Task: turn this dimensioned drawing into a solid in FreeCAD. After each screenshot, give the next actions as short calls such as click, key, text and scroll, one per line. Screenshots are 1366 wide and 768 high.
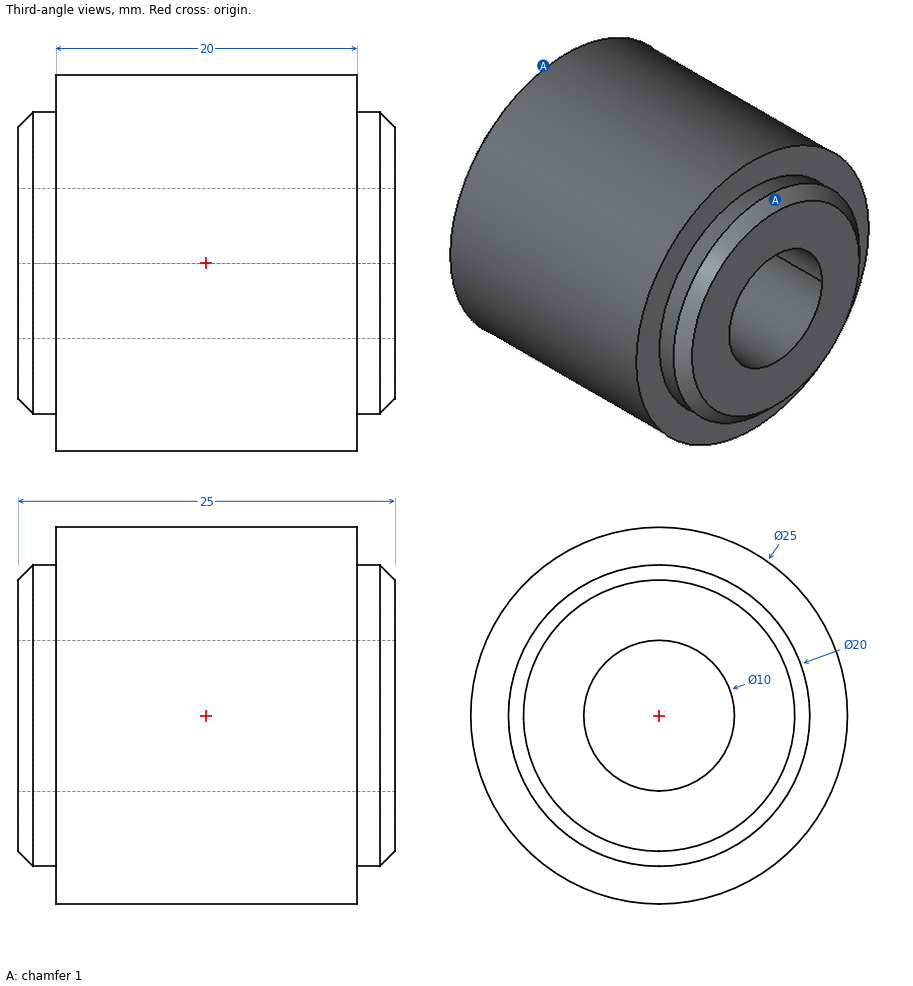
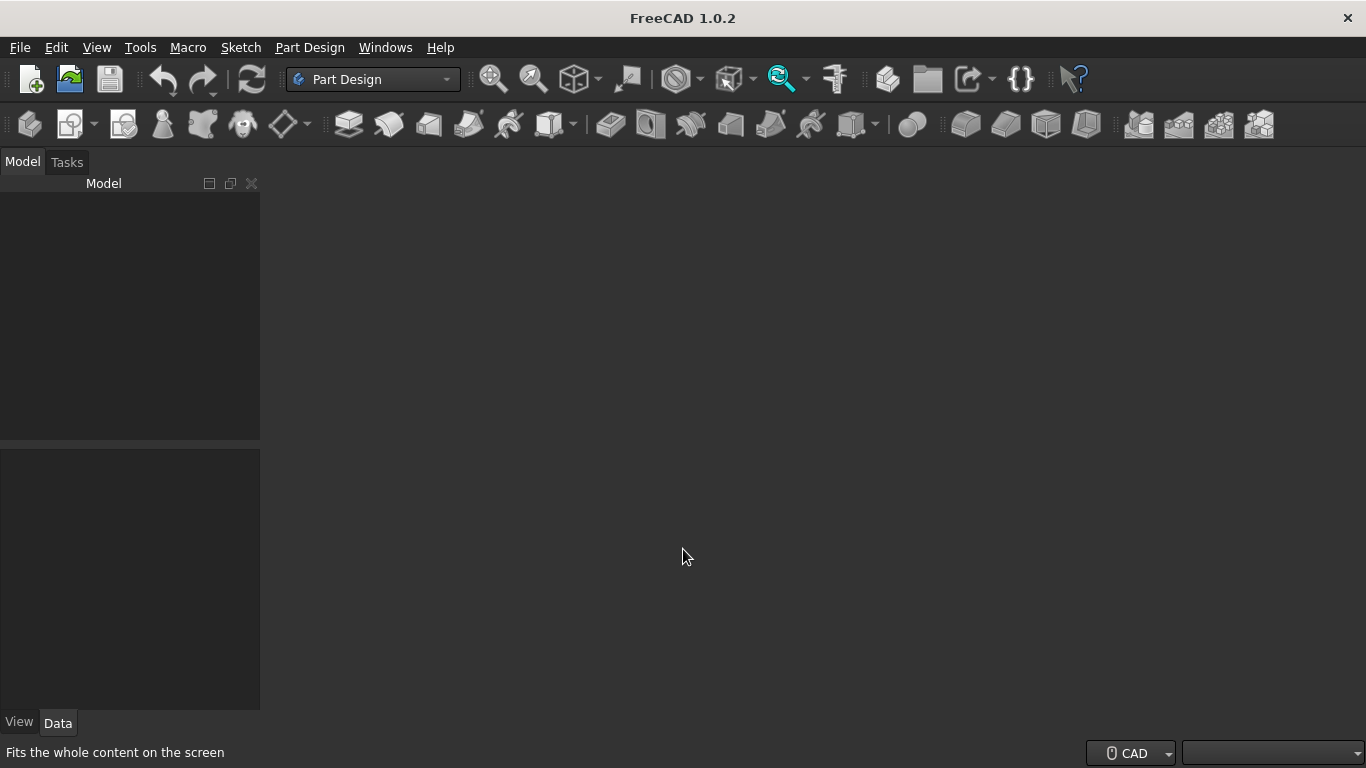
click(30, 80)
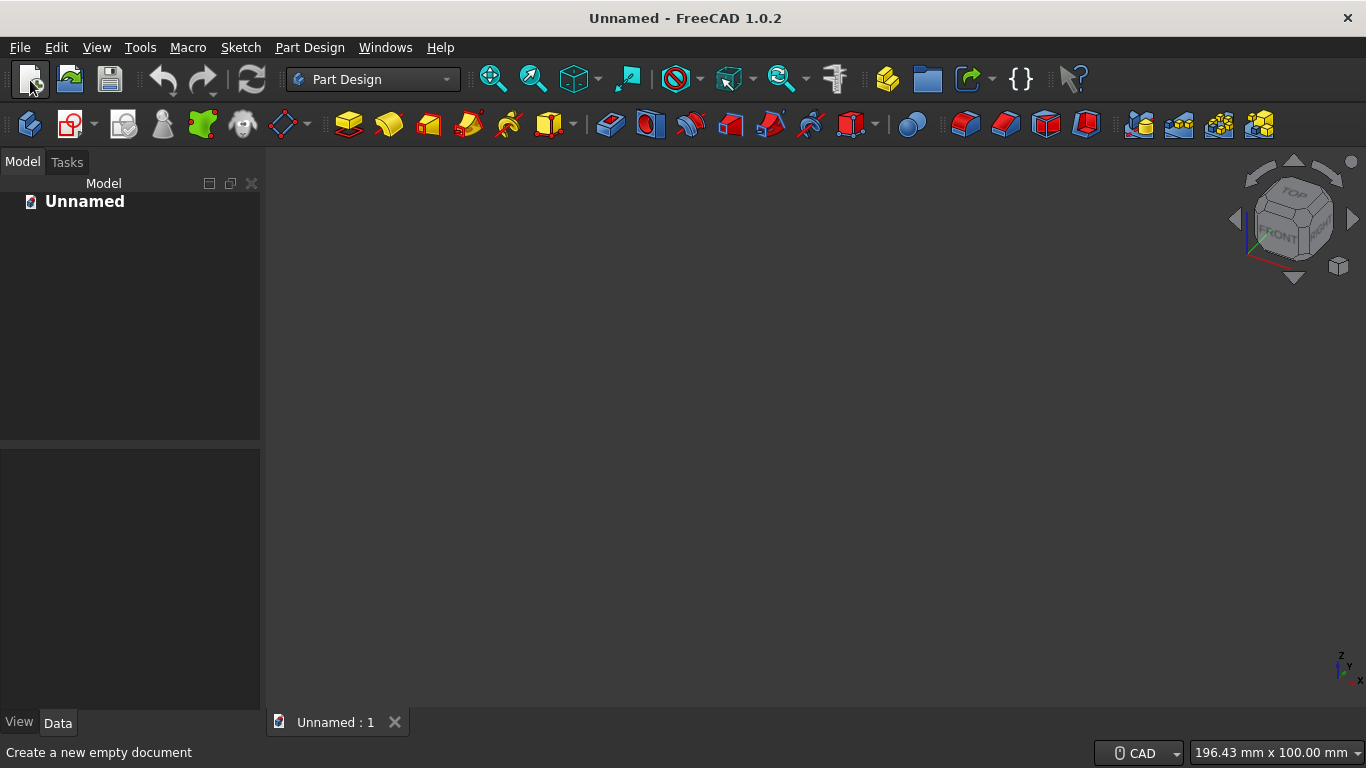
click(70, 124)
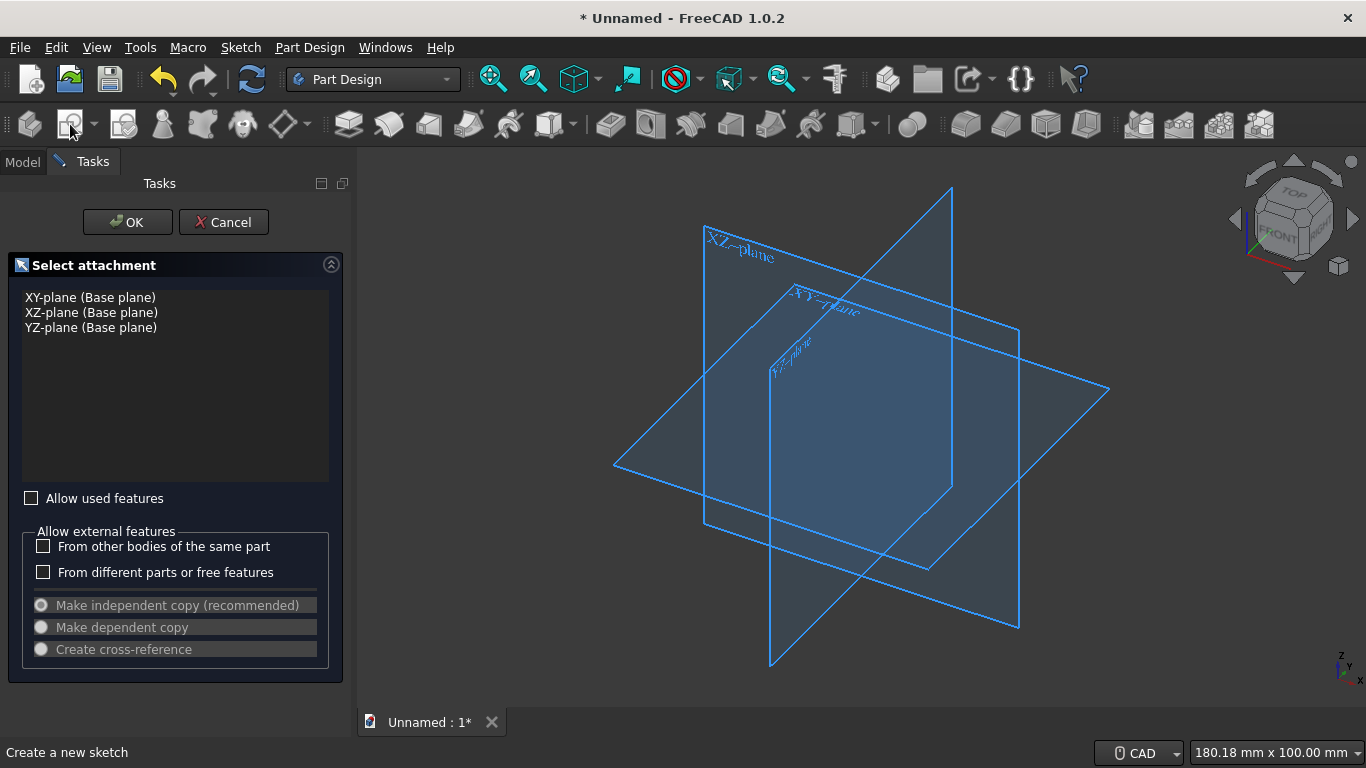
click(82, 328)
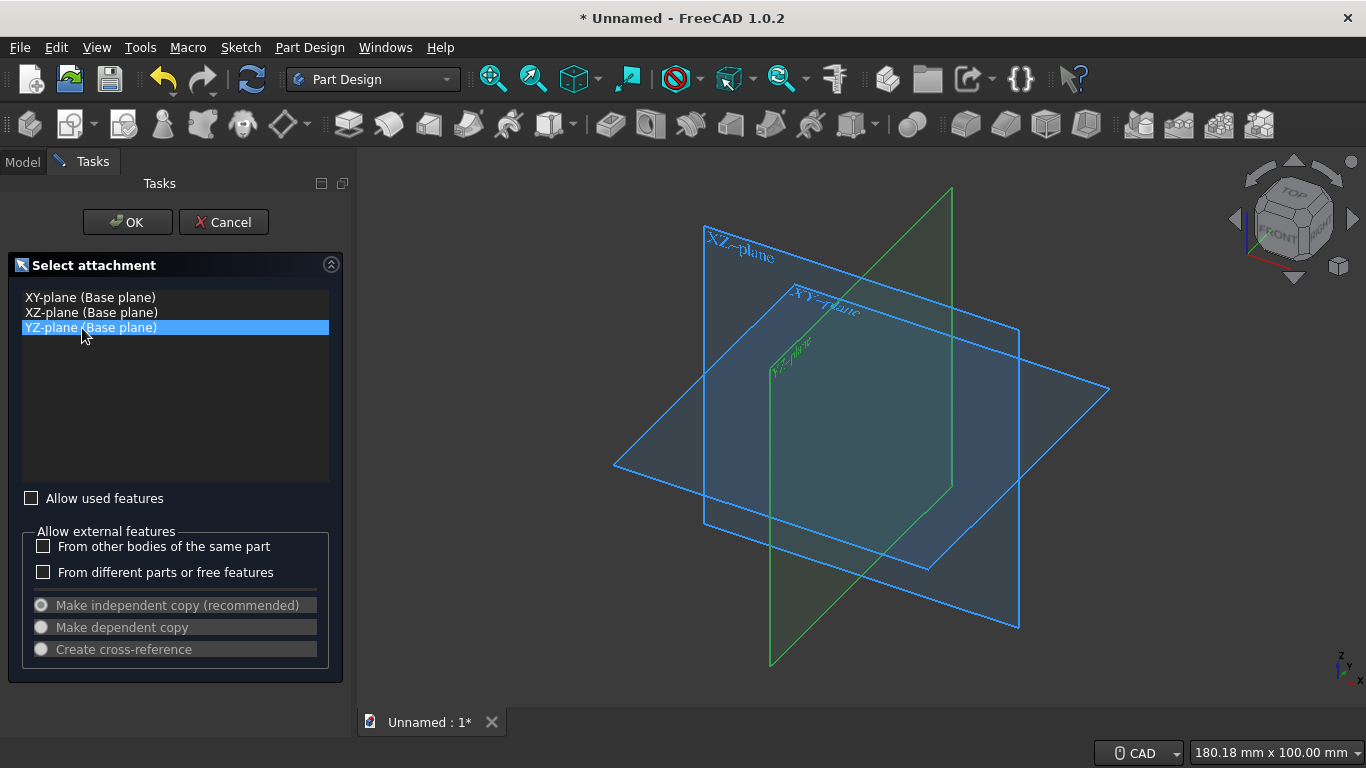
click(128, 222)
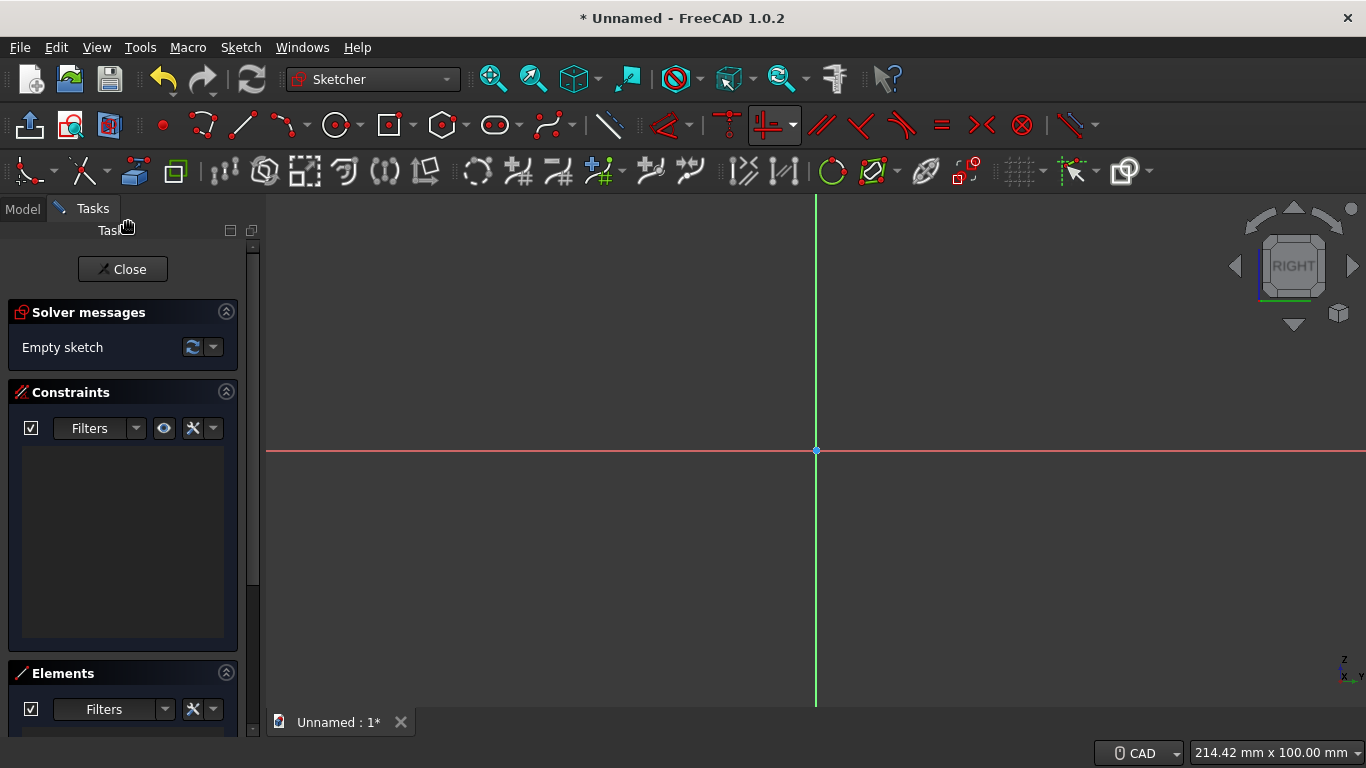
scroll(846, 450, up, 6)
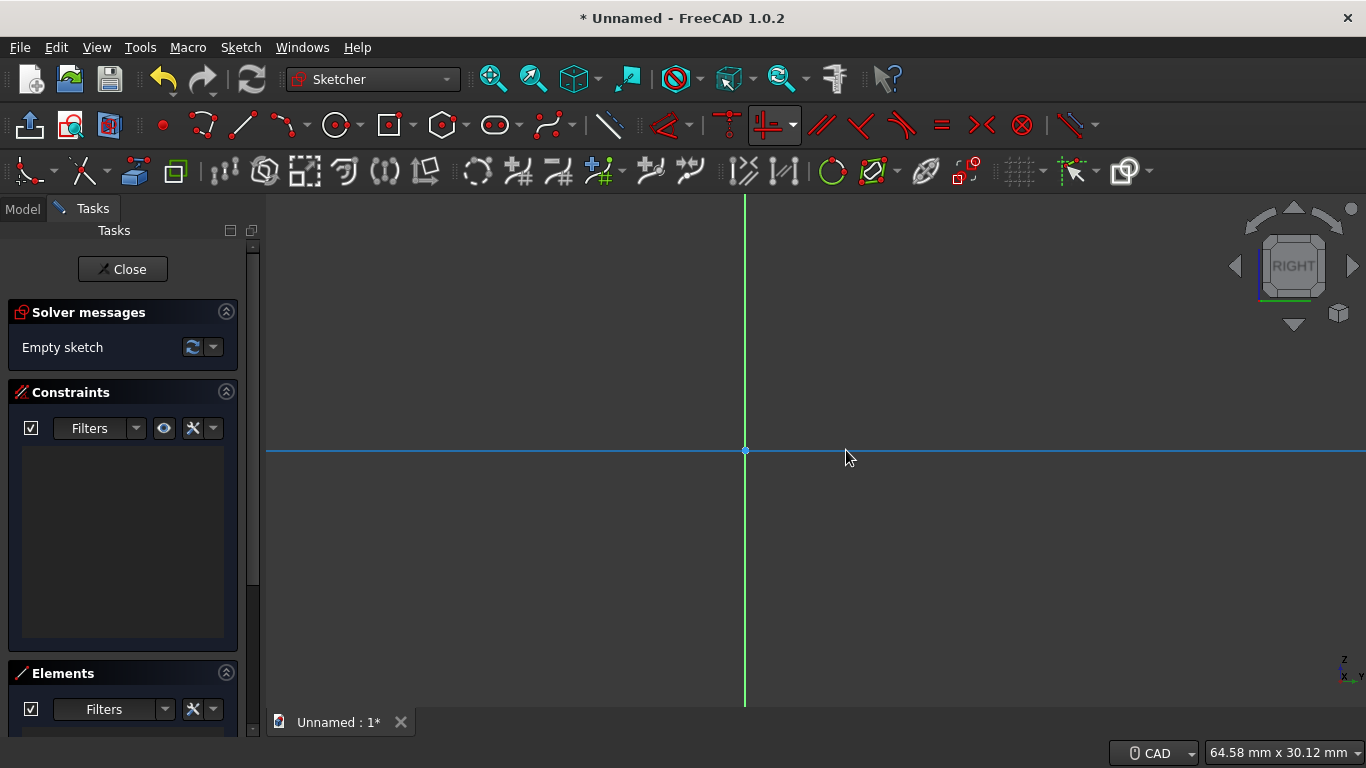
key(g)
key(c)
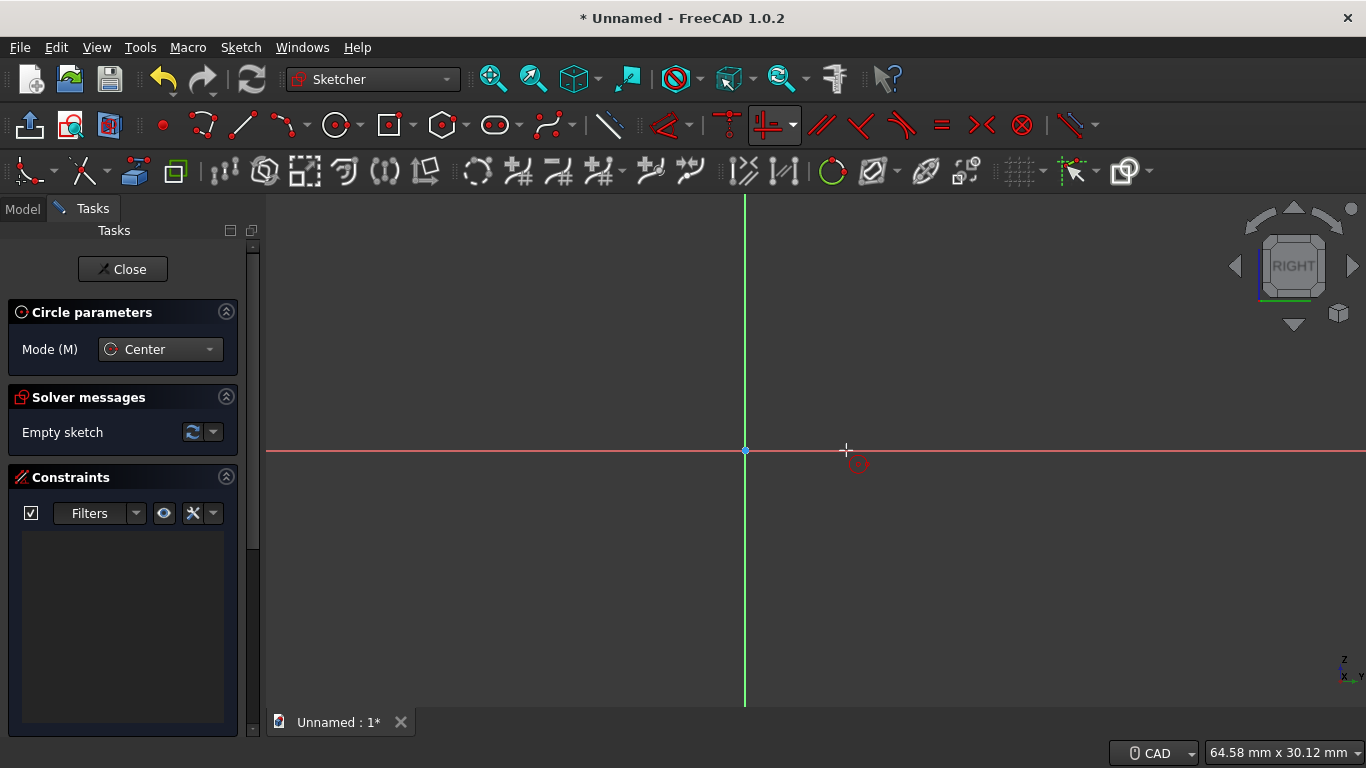
click(745, 450)
move(866, 330)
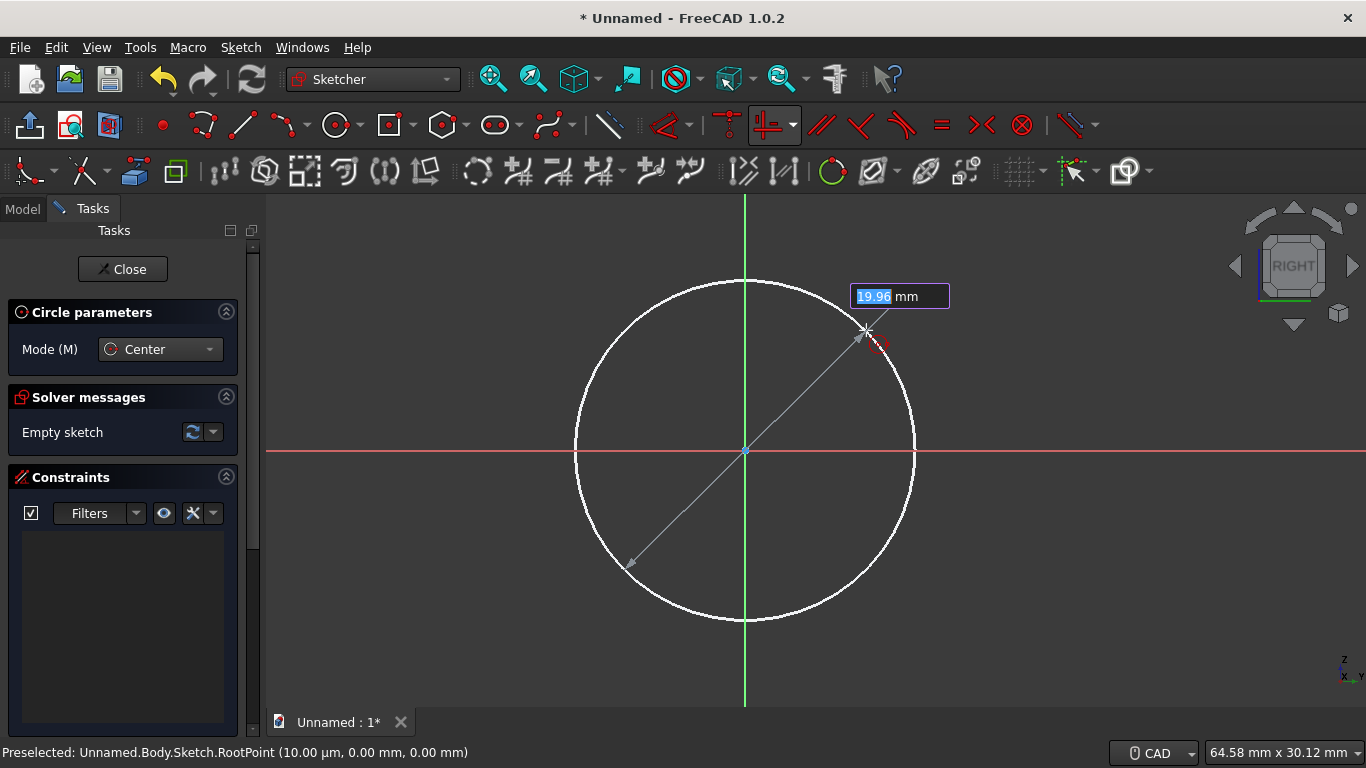
text(20)
key(Return)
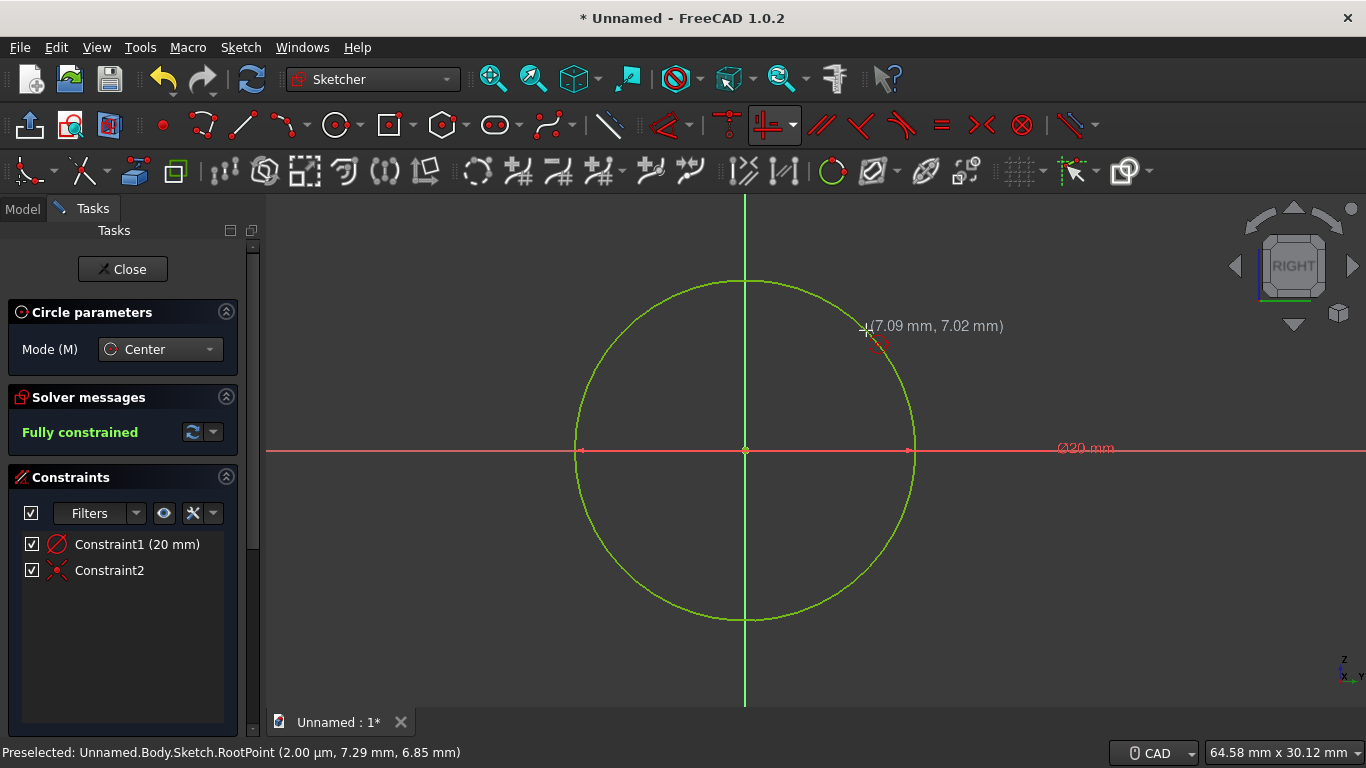
click(745, 450)
move(805, 390)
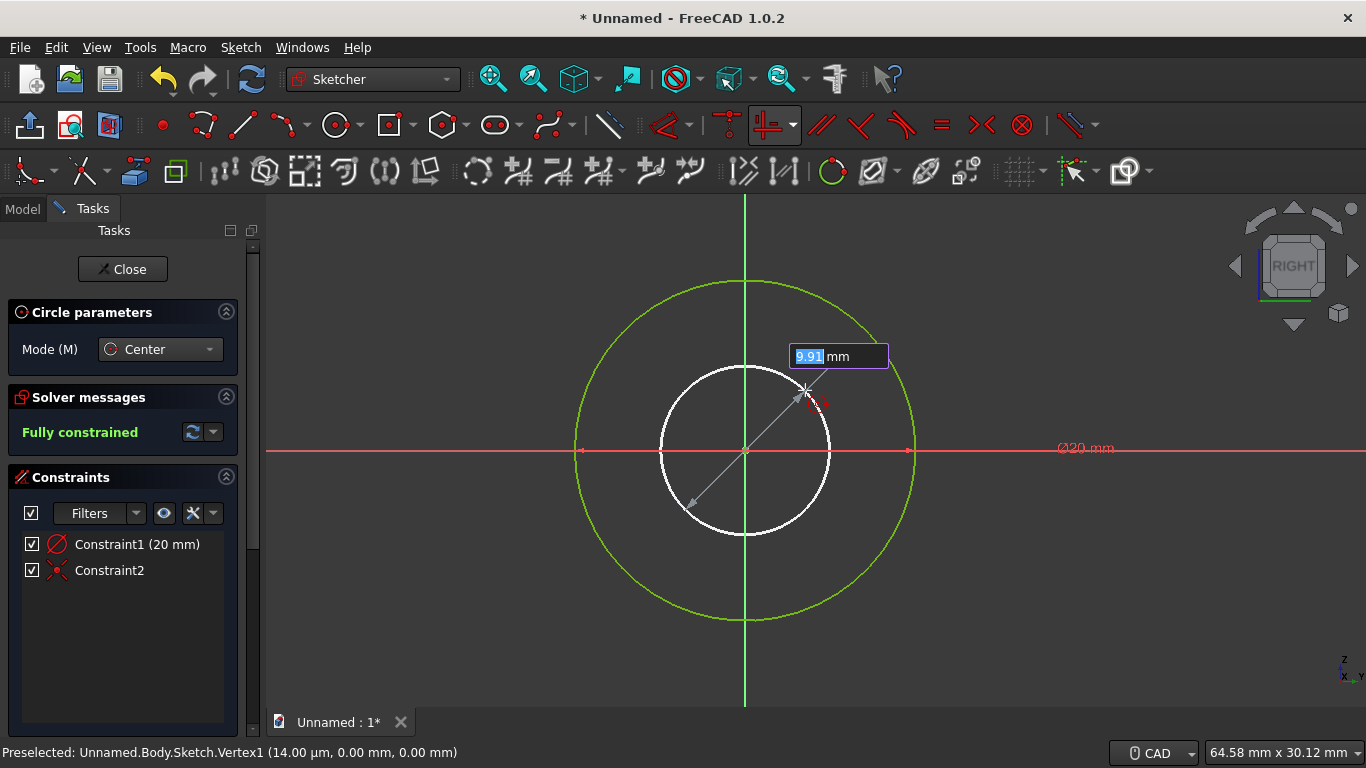
text(10)
key(Return)
key(Escape)